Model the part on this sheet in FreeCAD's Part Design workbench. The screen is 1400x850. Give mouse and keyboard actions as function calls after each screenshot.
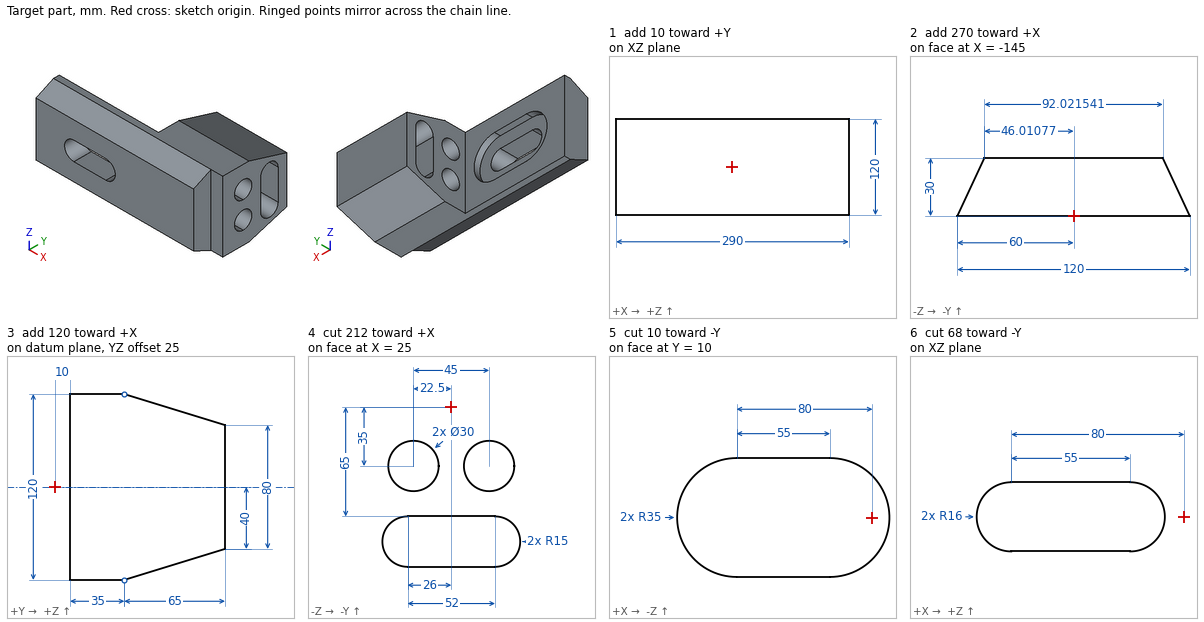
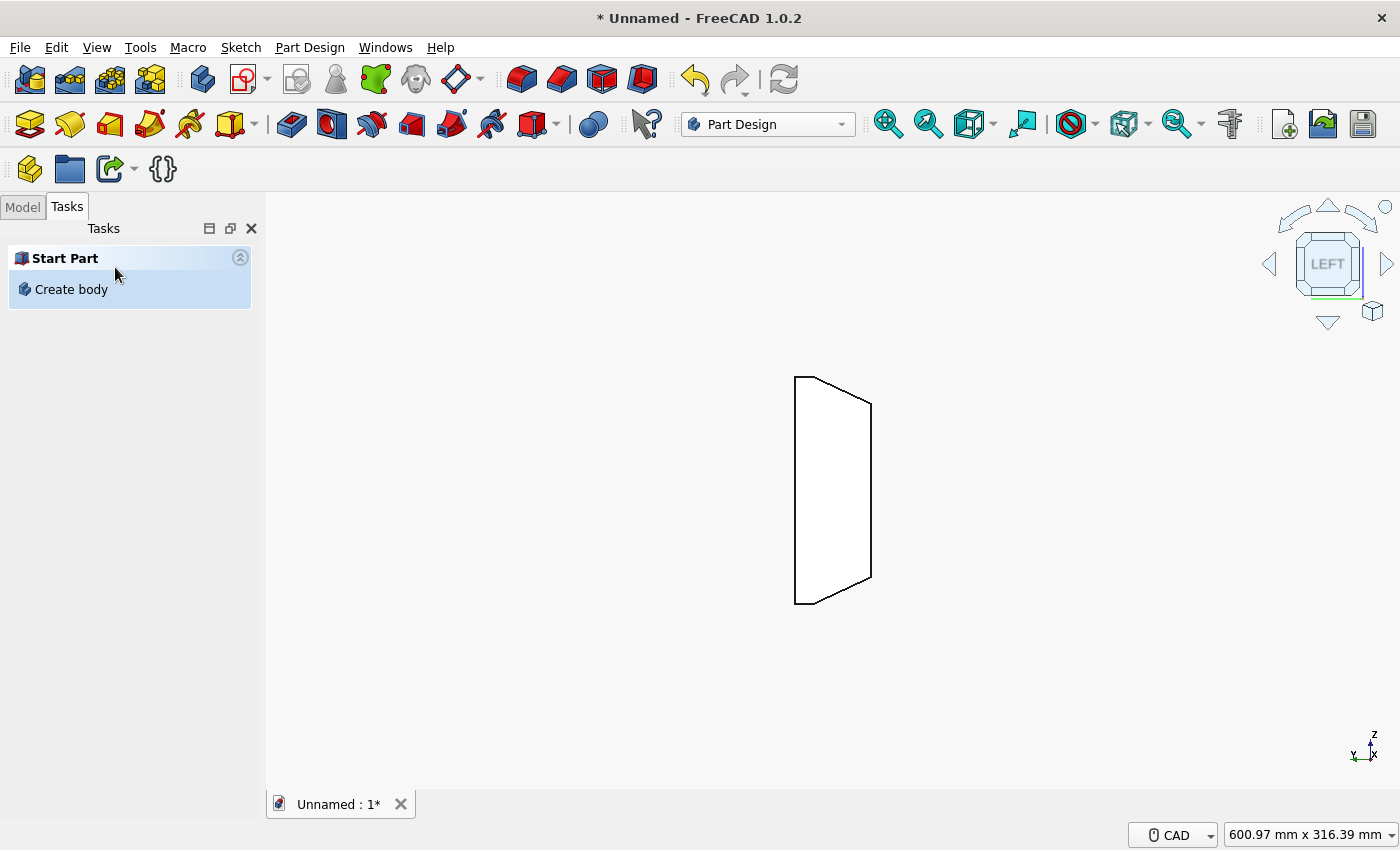
click(23, 206)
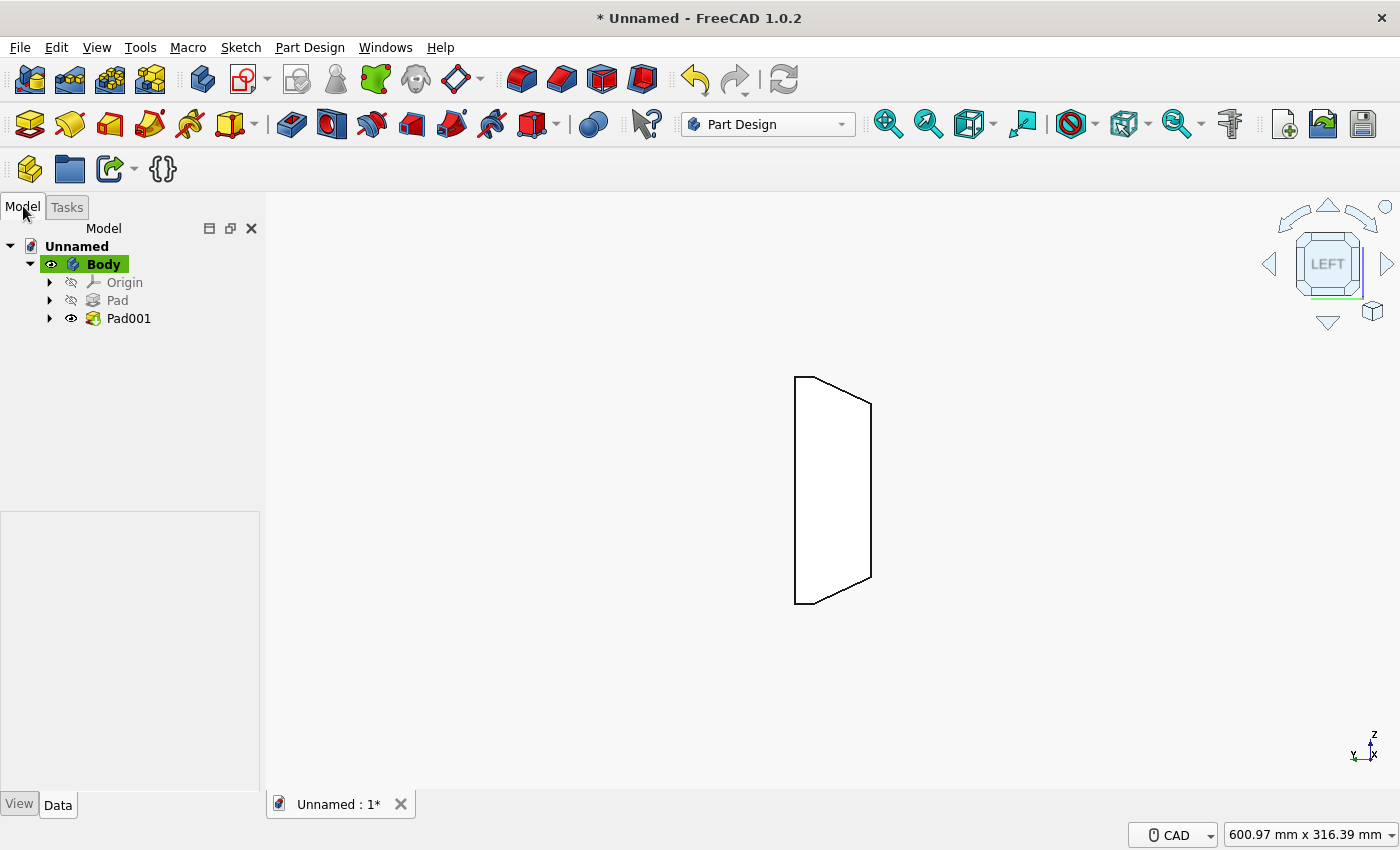
click(50, 282)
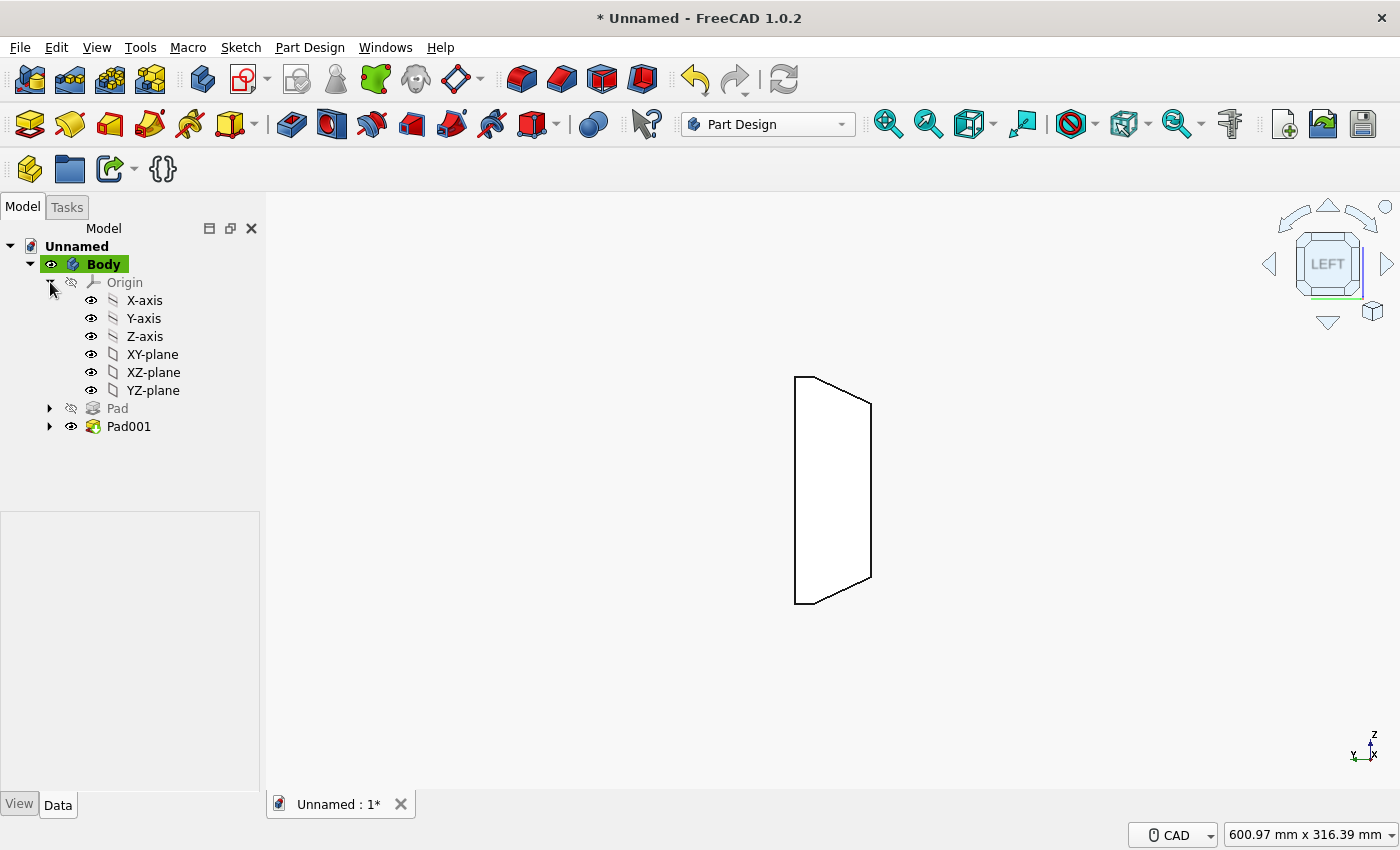
click(136, 390)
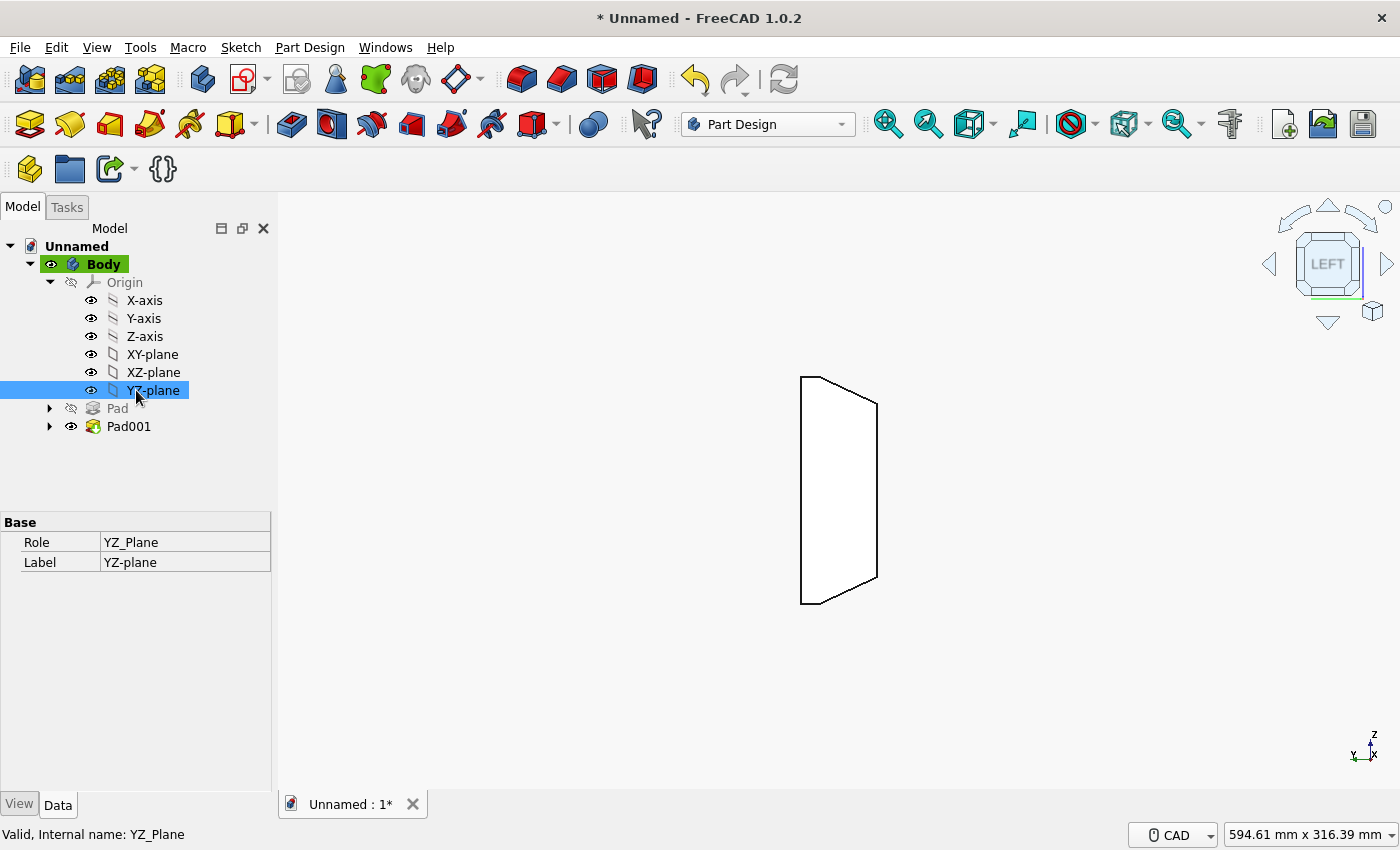
click(456, 80)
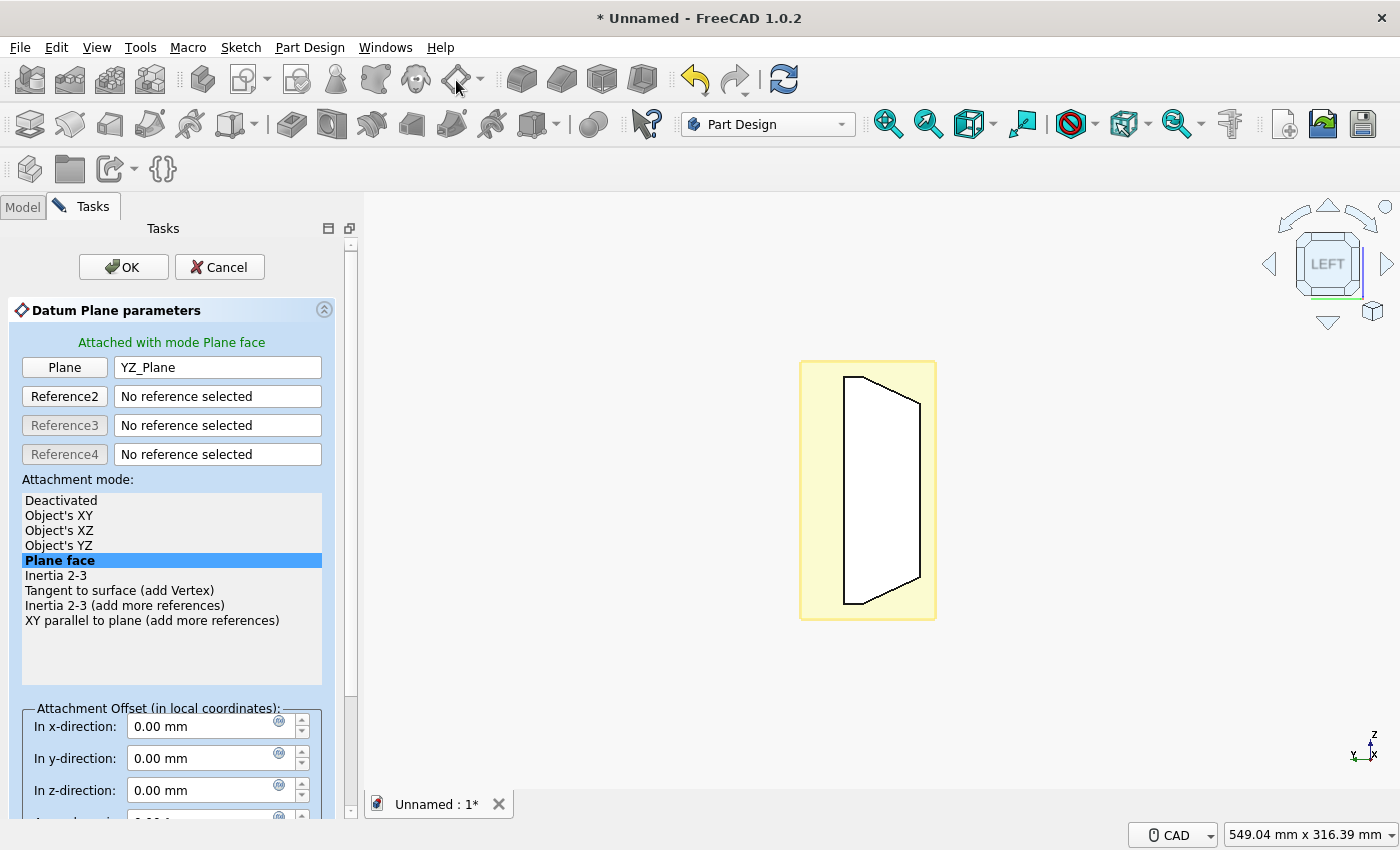
triple_click(210, 790)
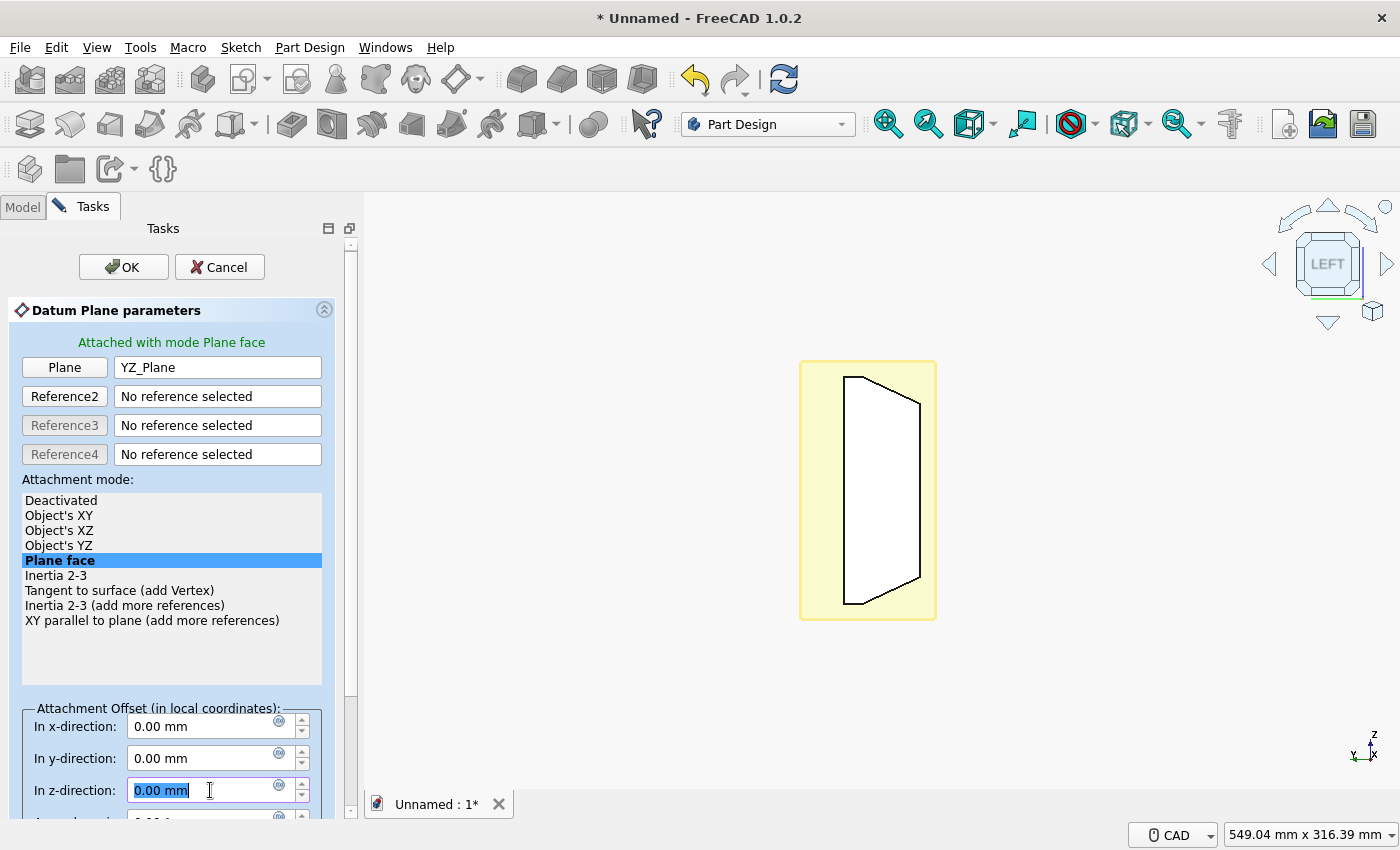
text(25)
key(Tab)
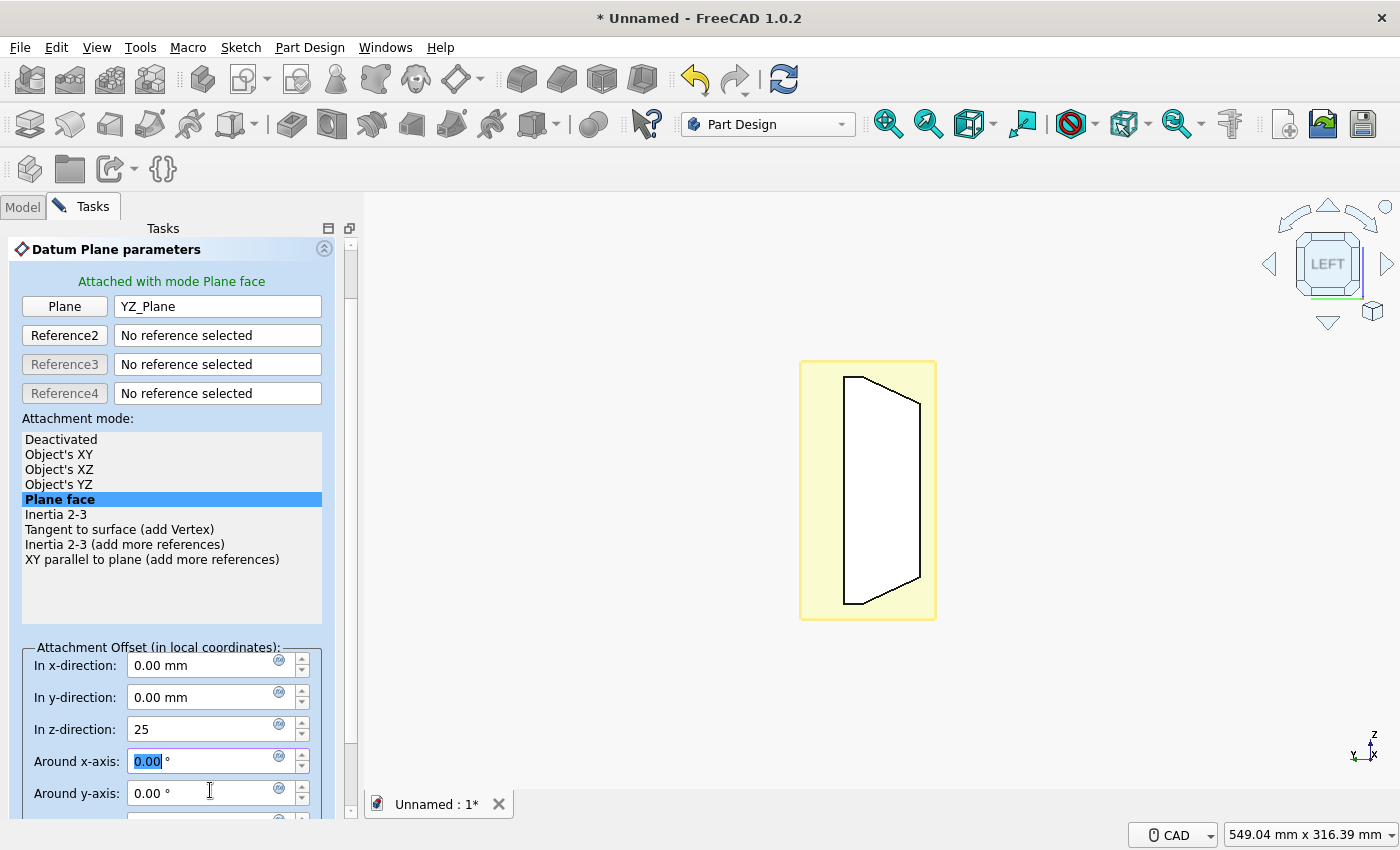
scroll(351, 528, up, 2)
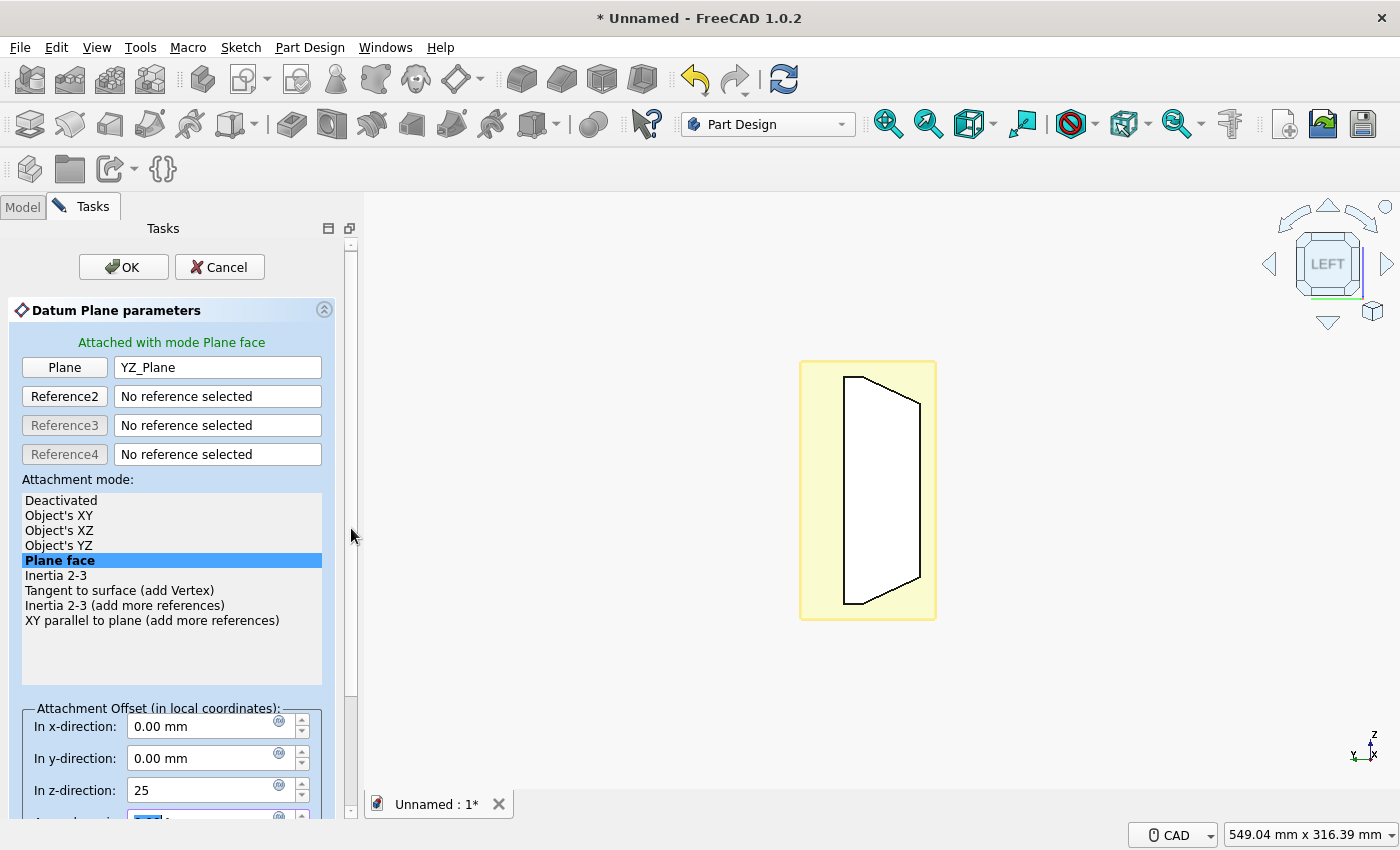
click(124, 267)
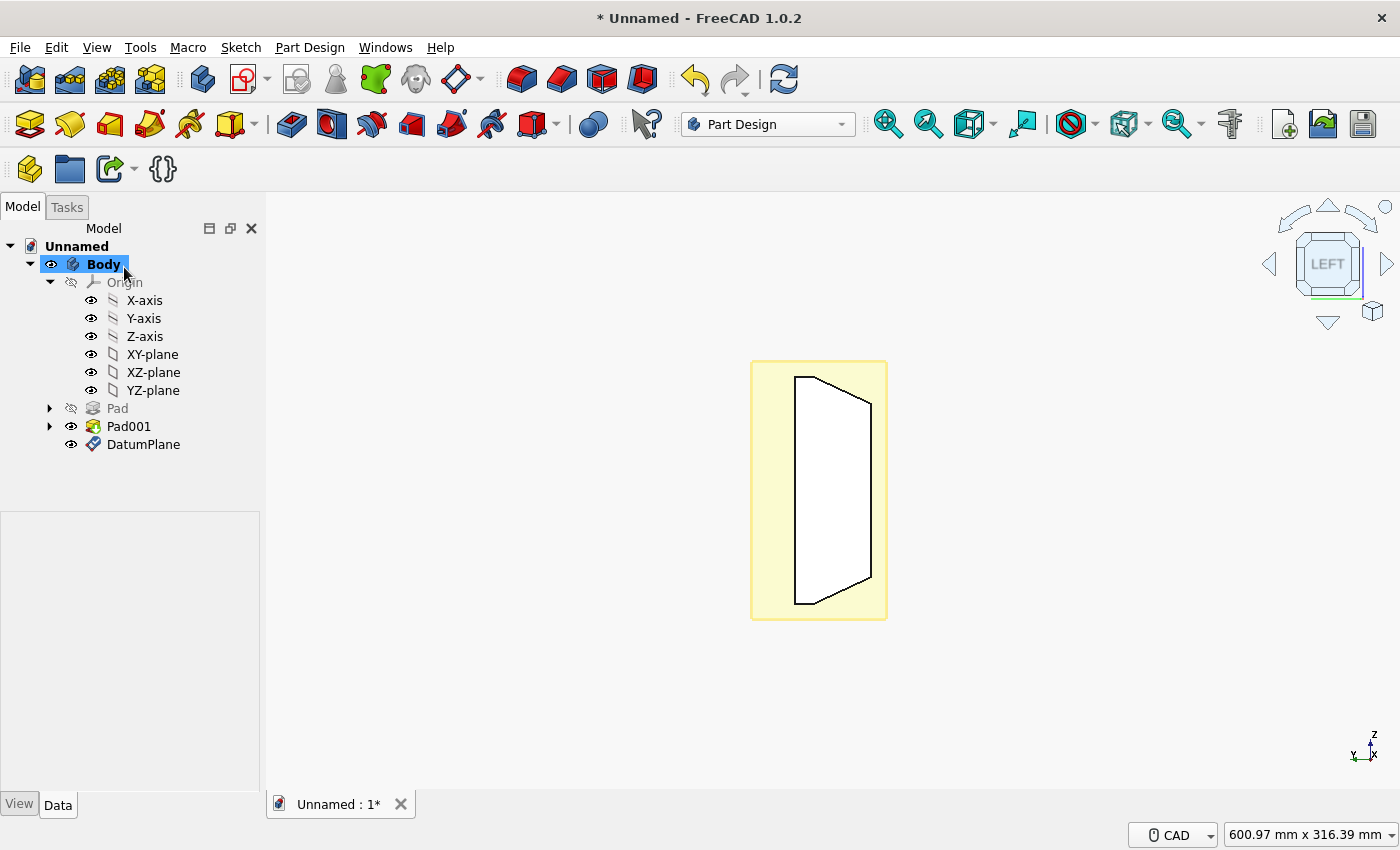
click(116, 444)